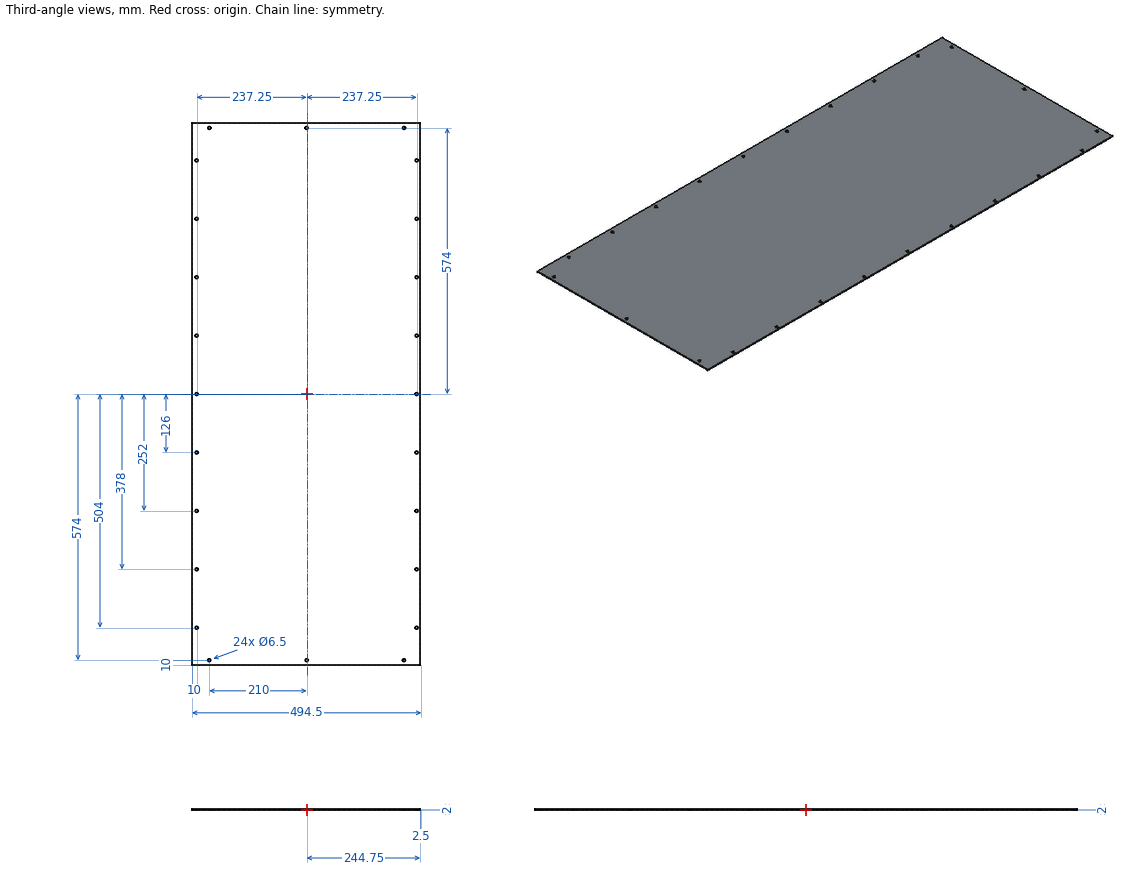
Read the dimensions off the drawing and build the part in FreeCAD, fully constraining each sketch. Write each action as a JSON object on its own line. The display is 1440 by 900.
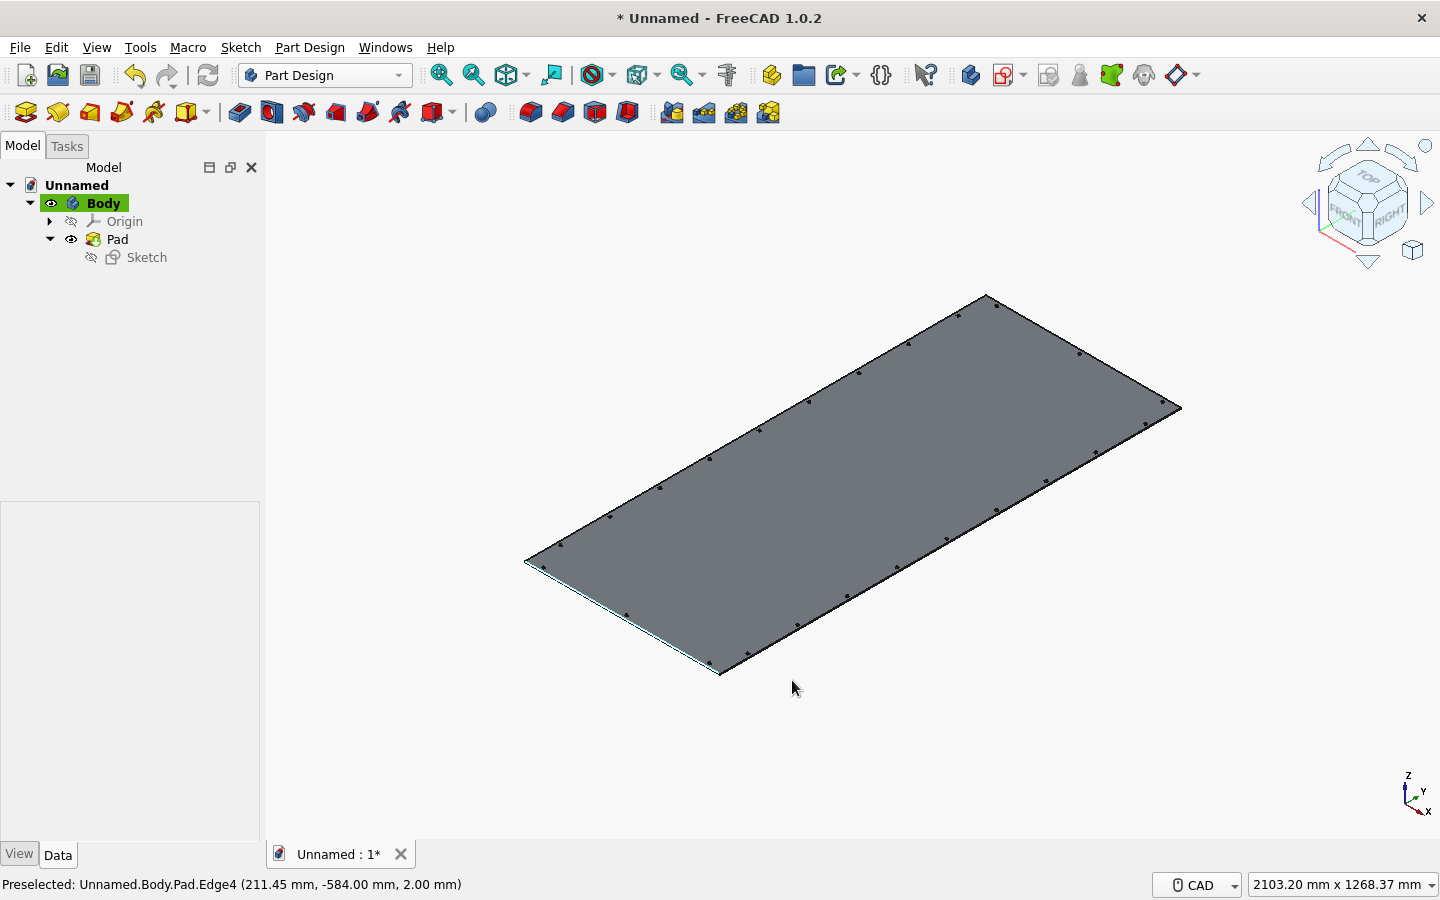
{"action": "scroll", "coordinate": [706, 665], "scroll_direction": "up", "scroll_amount": 15}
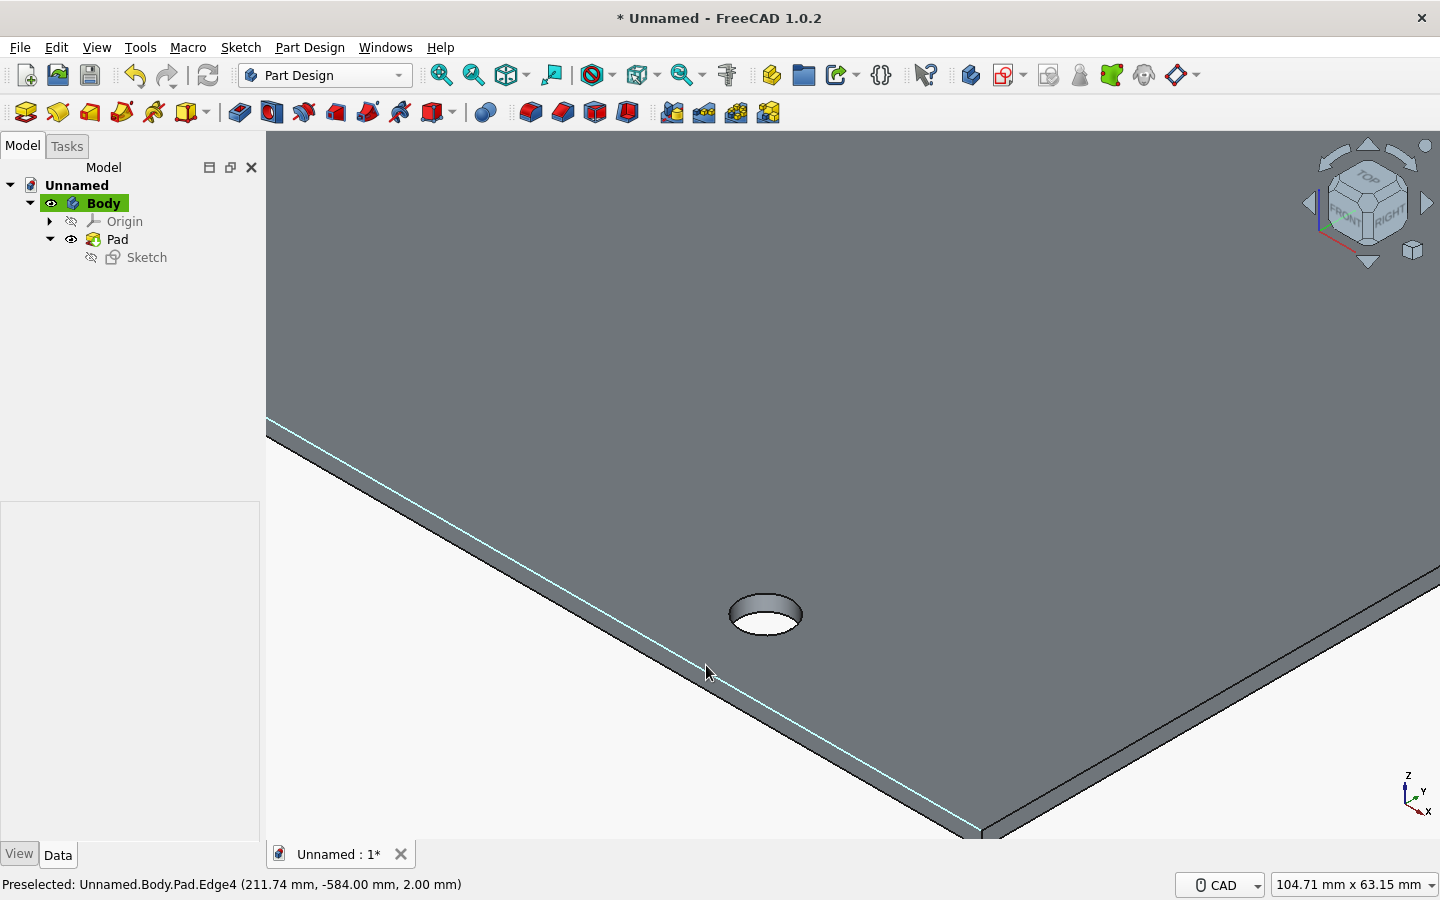
{"action": "key", "text": "v f"}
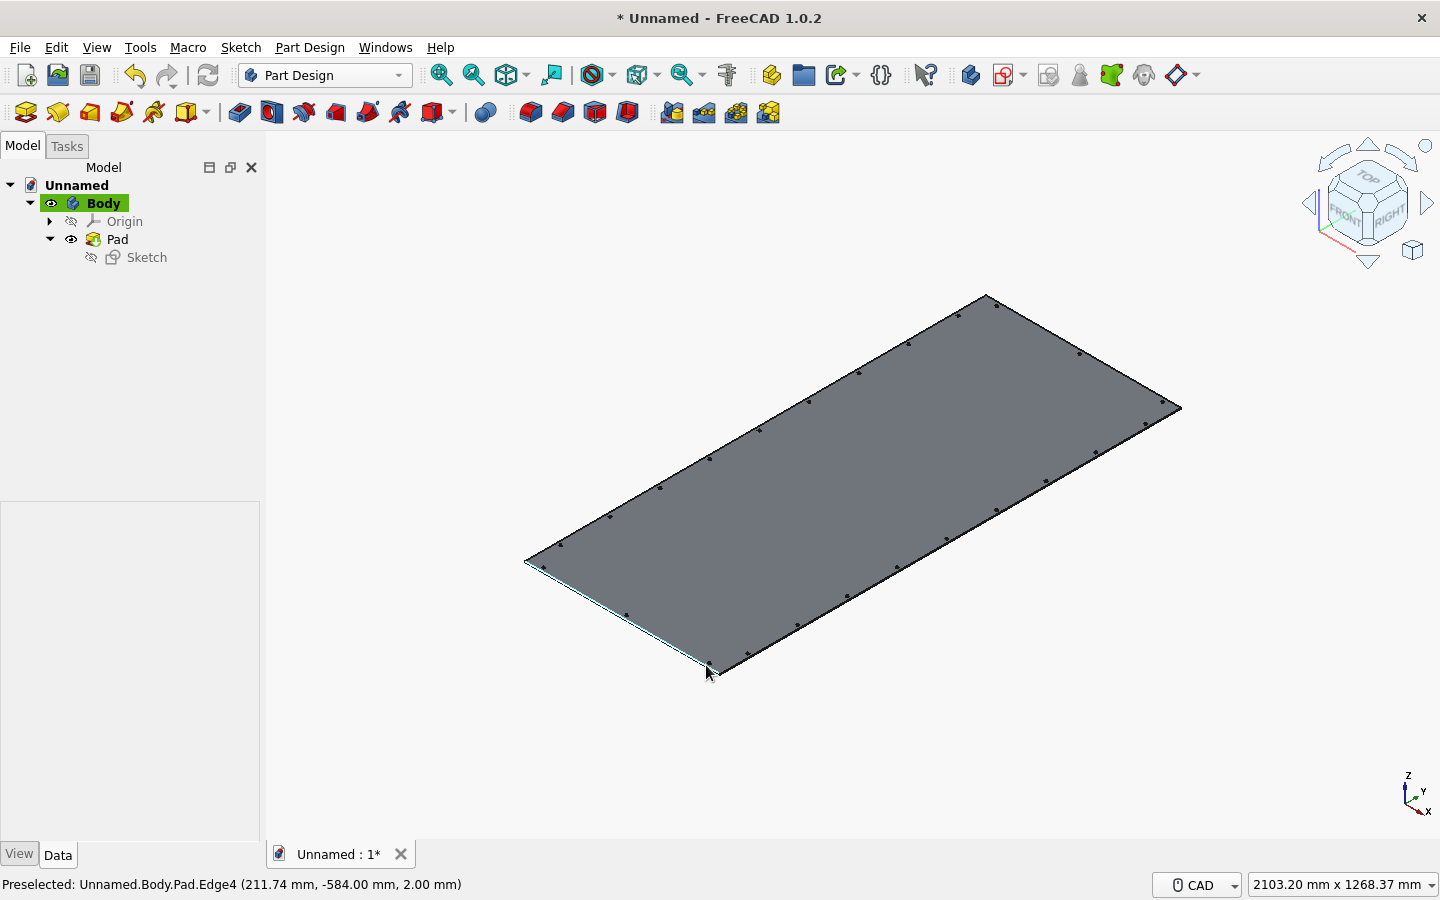
{"action": "key", "text": "1"}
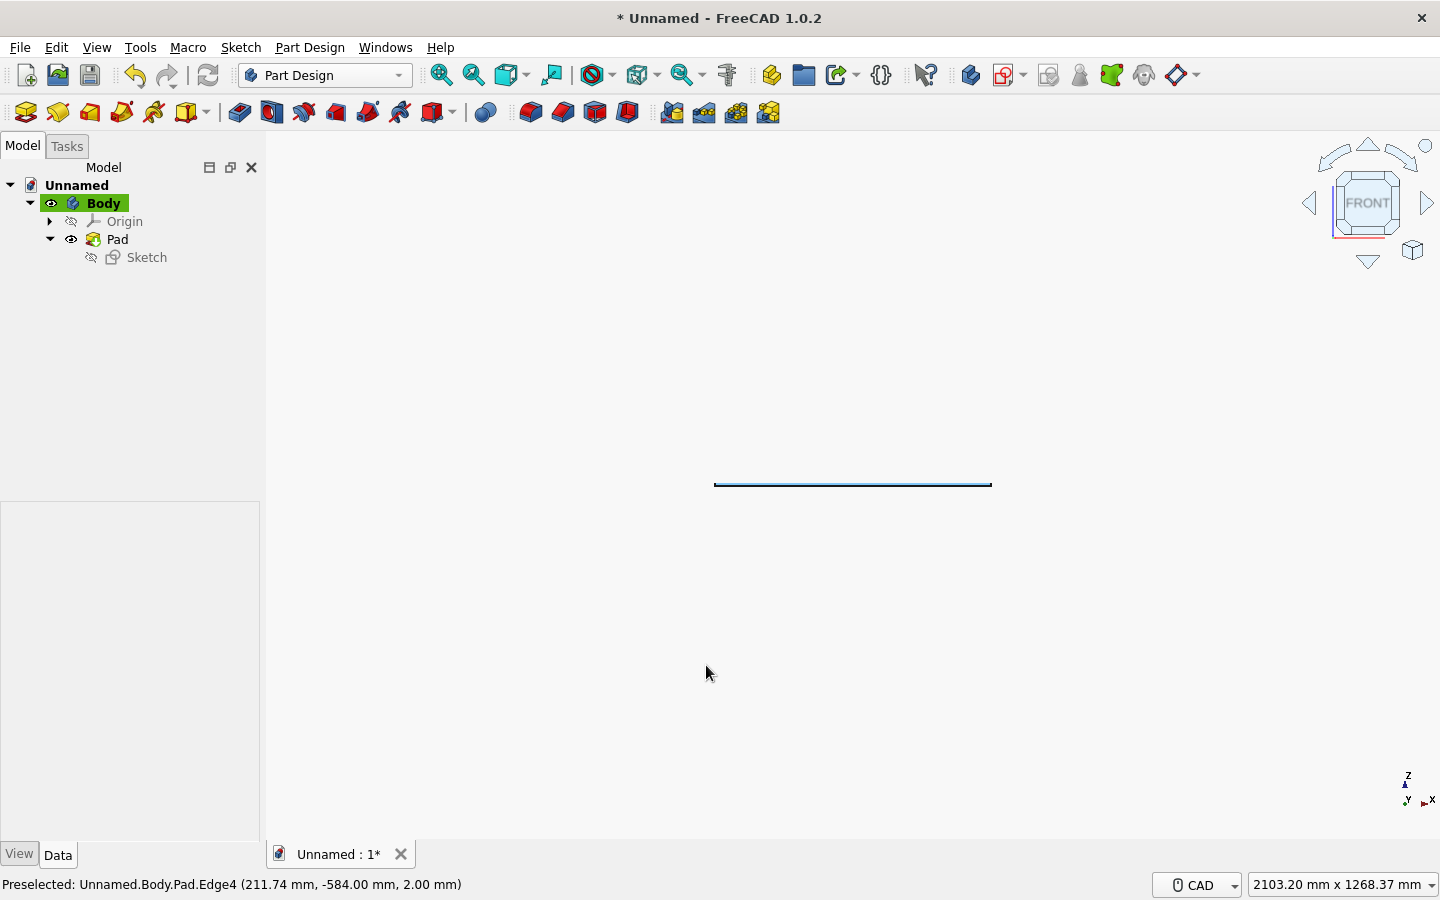
{"action": "key", "text": "v f"}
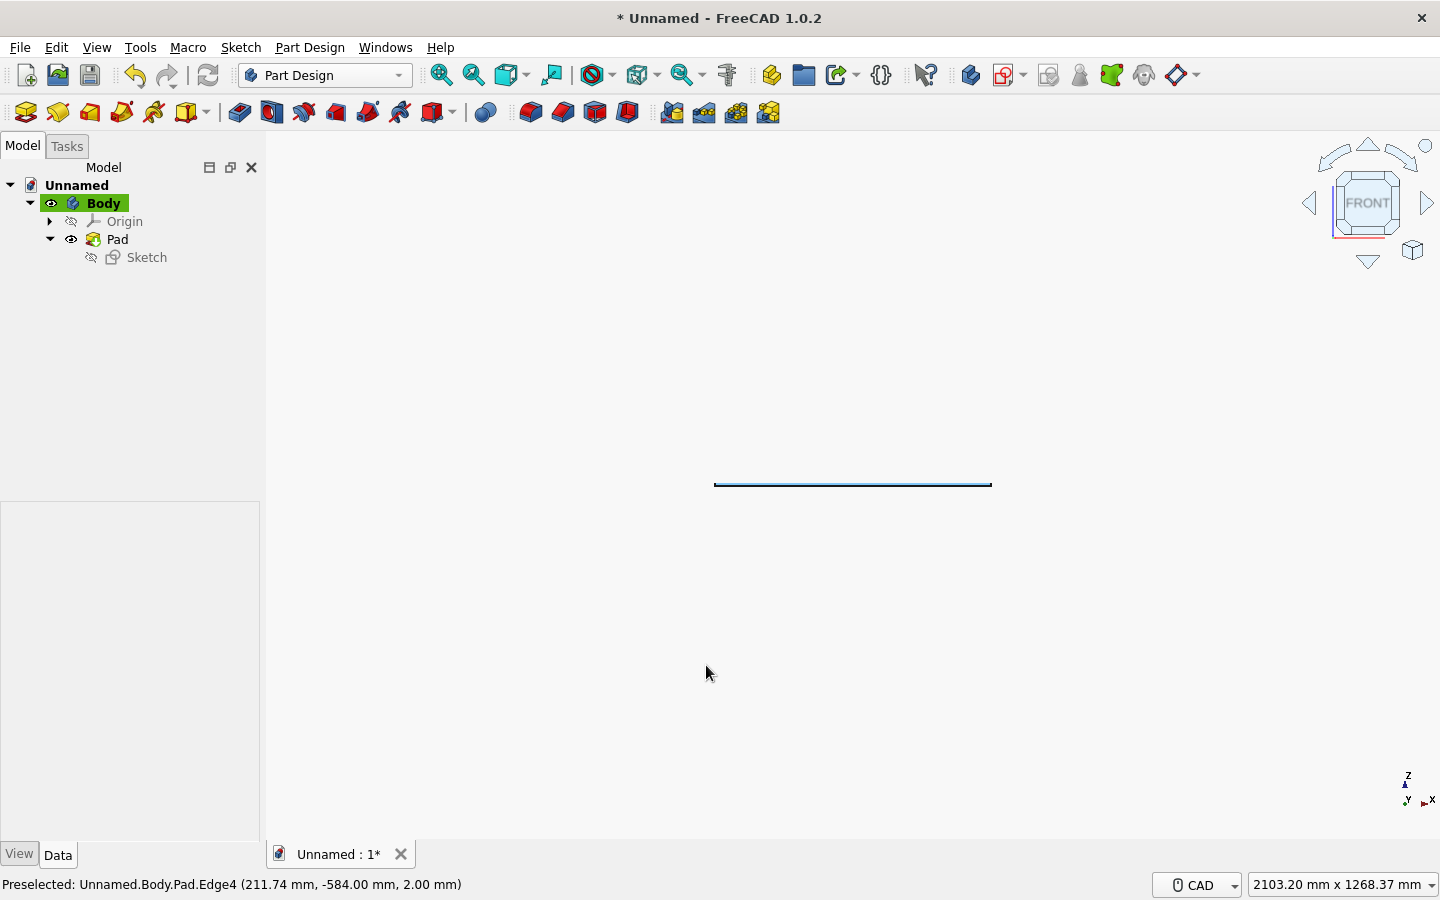
{"action": "scroll", "coordinate": [971, 484], "scroll_direction": "up", "scroll_amount": 15}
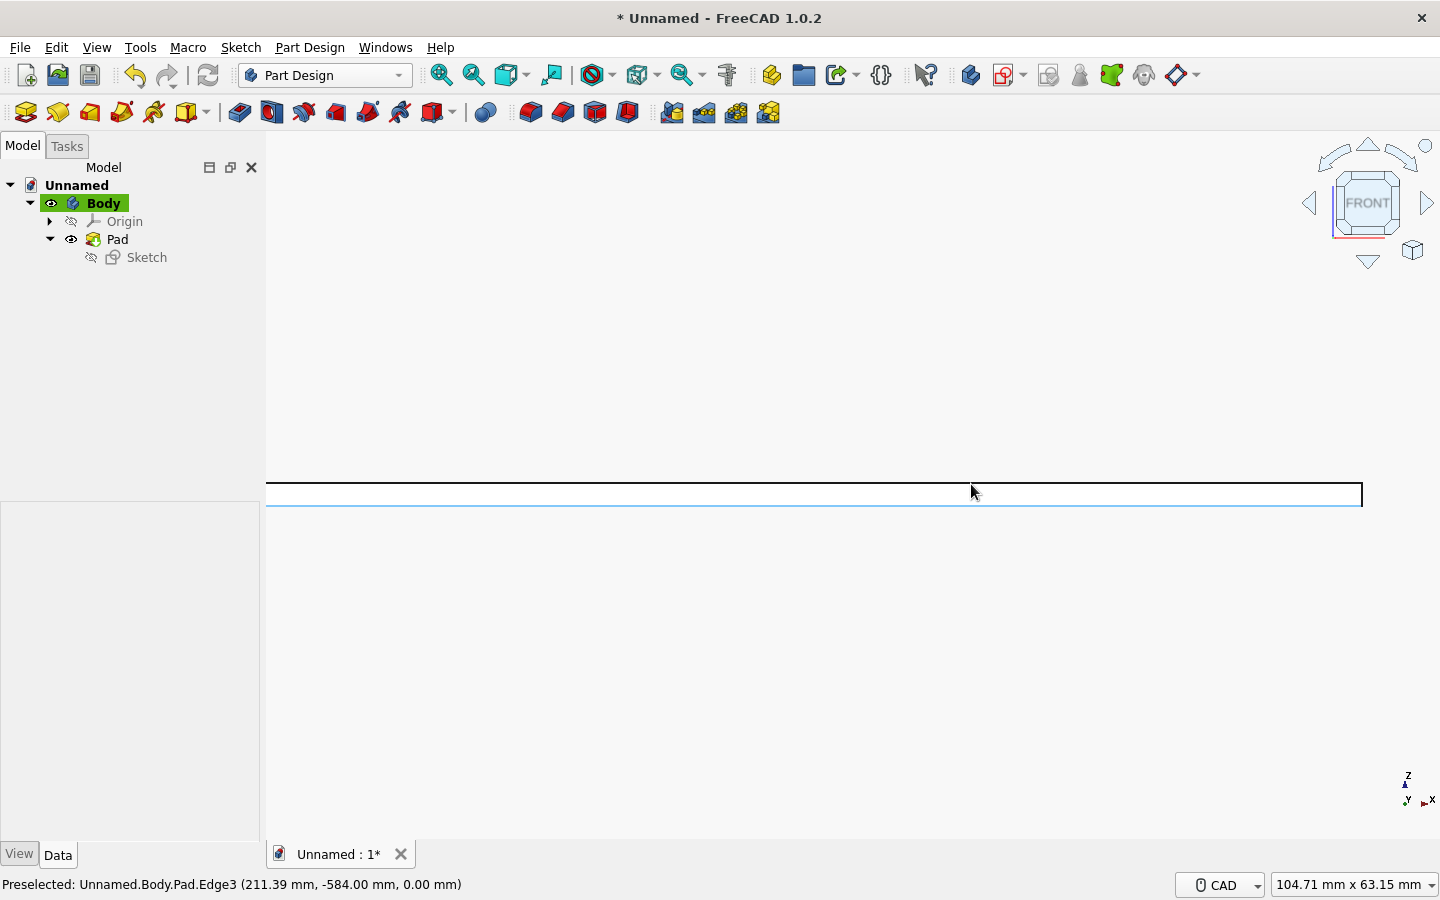
{"action": "left_click", "coordinate": [966, 494]}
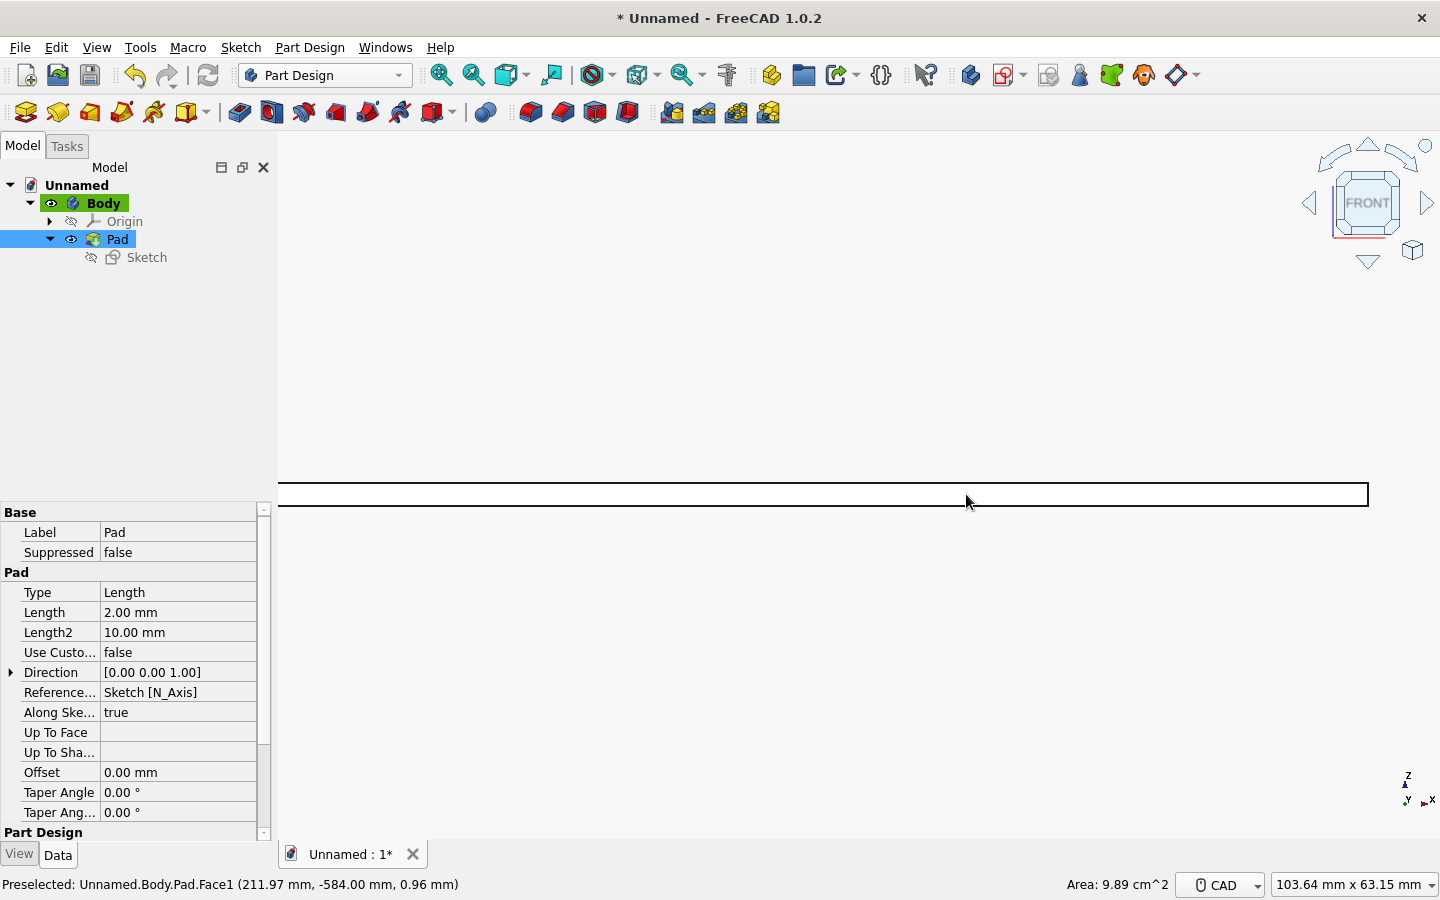
{"action": "left_click", "coordinate": [1004, 76]}